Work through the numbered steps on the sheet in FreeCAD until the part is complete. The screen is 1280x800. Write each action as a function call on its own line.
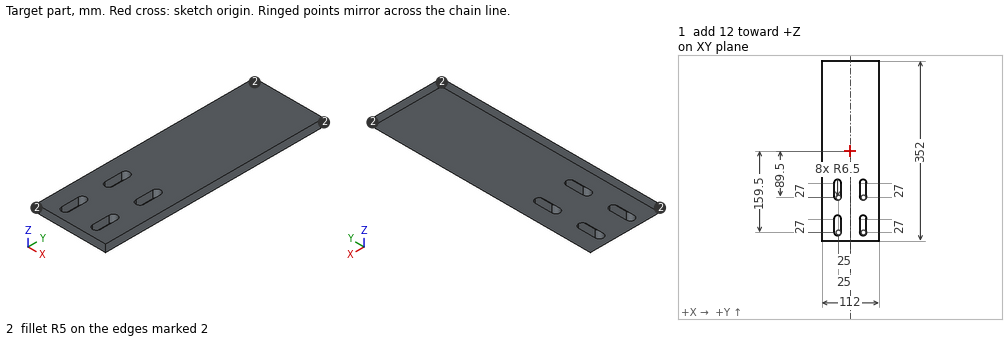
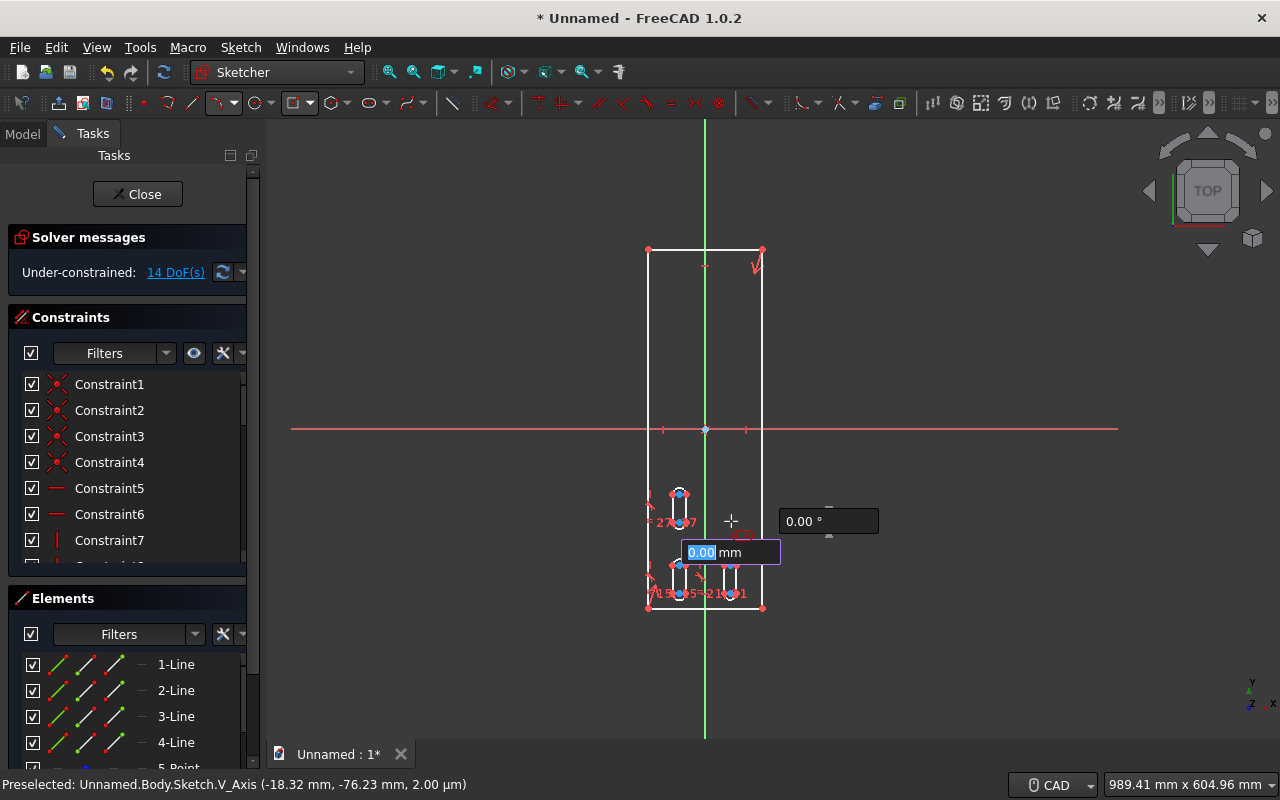
click(731, 493)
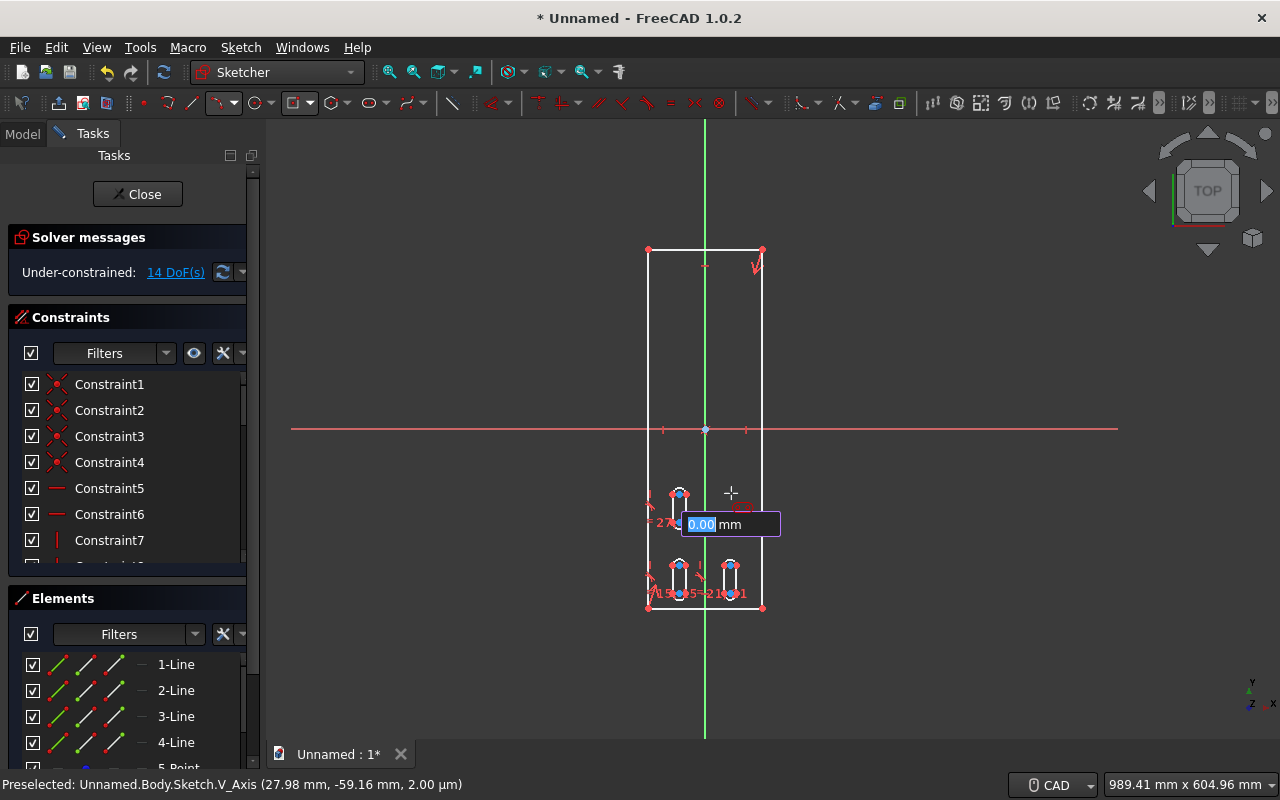
scroll(737, 507, up, 5)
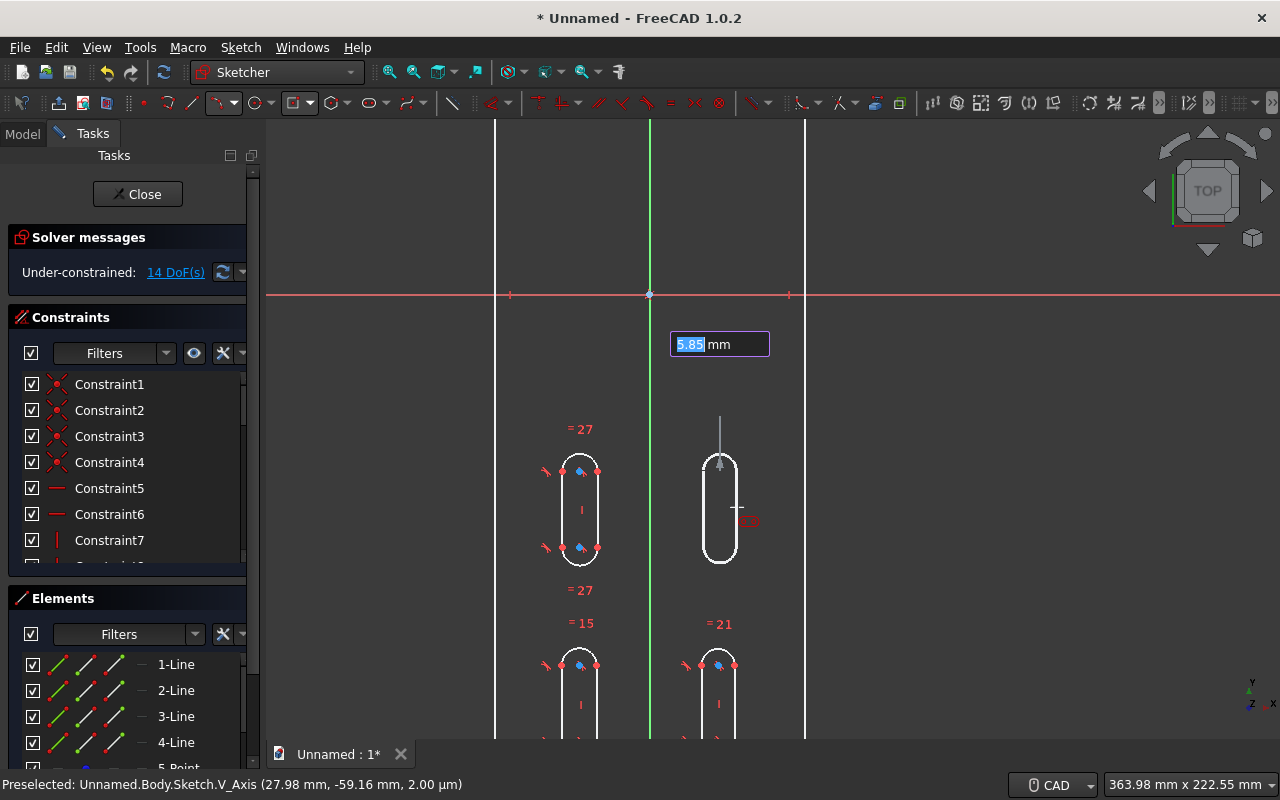
click(737, 506)
key(Escape)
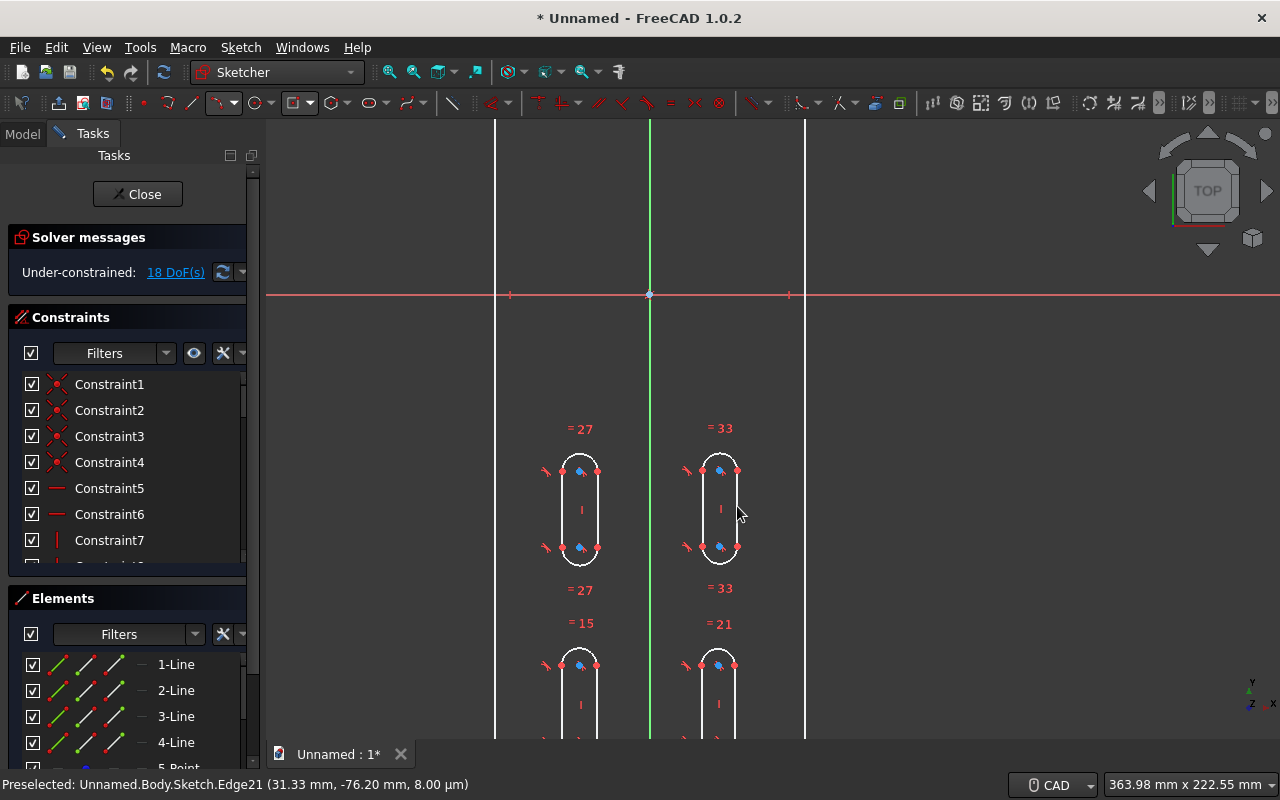
scroll(736, 507, down, 5)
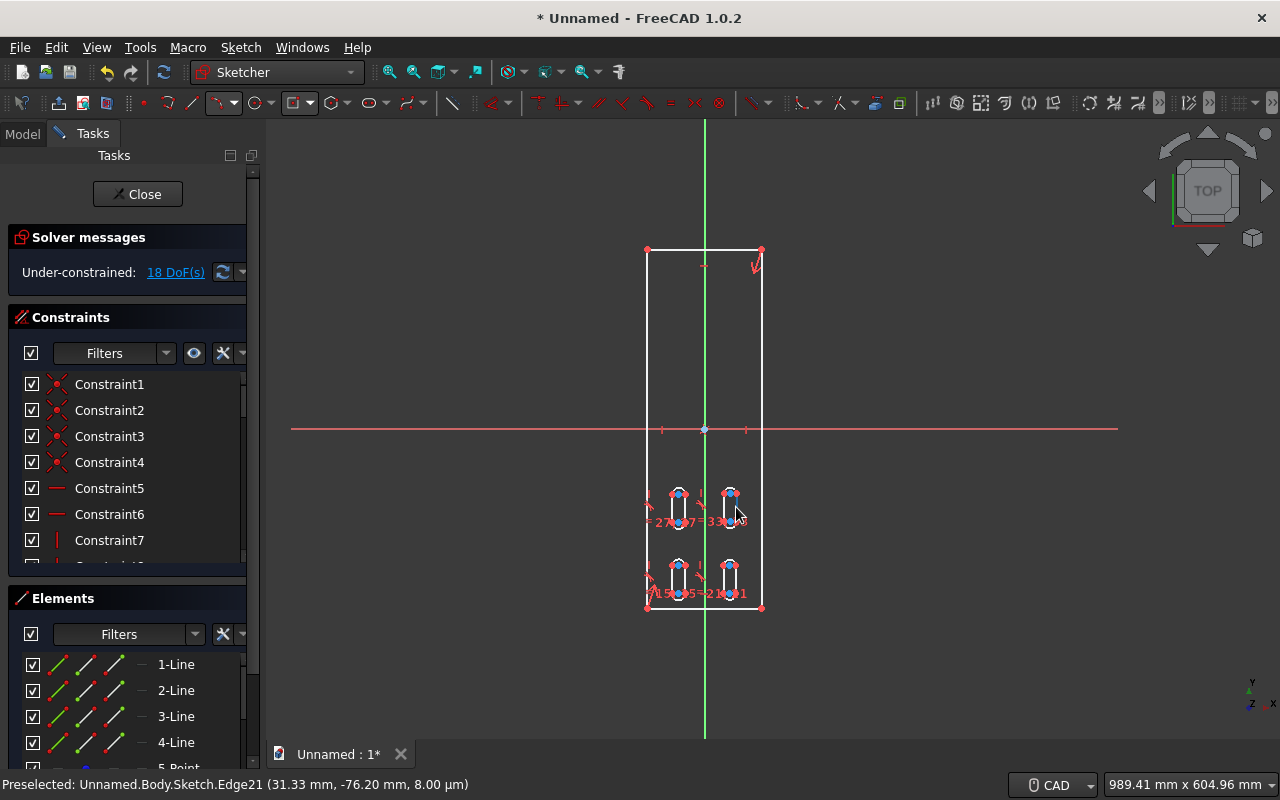
scroll(675, 599, up, 5)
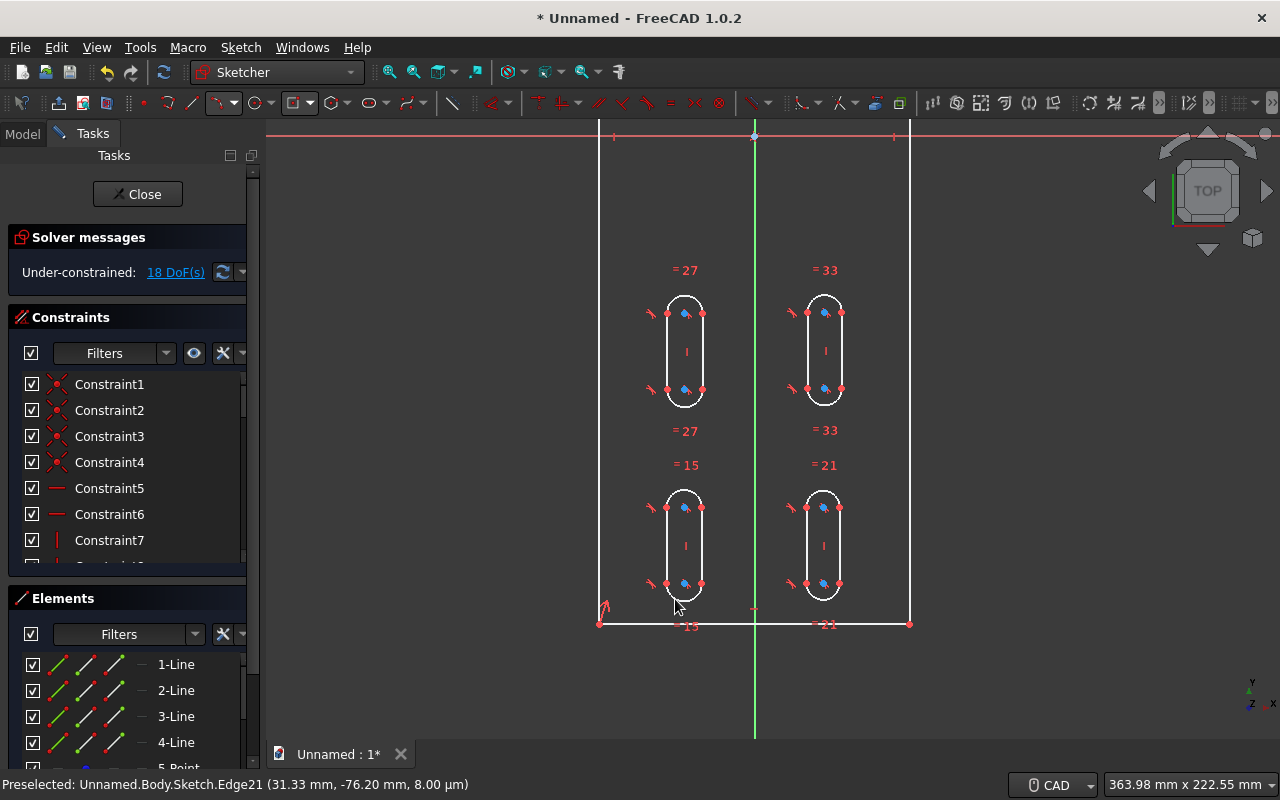
click(674, 598)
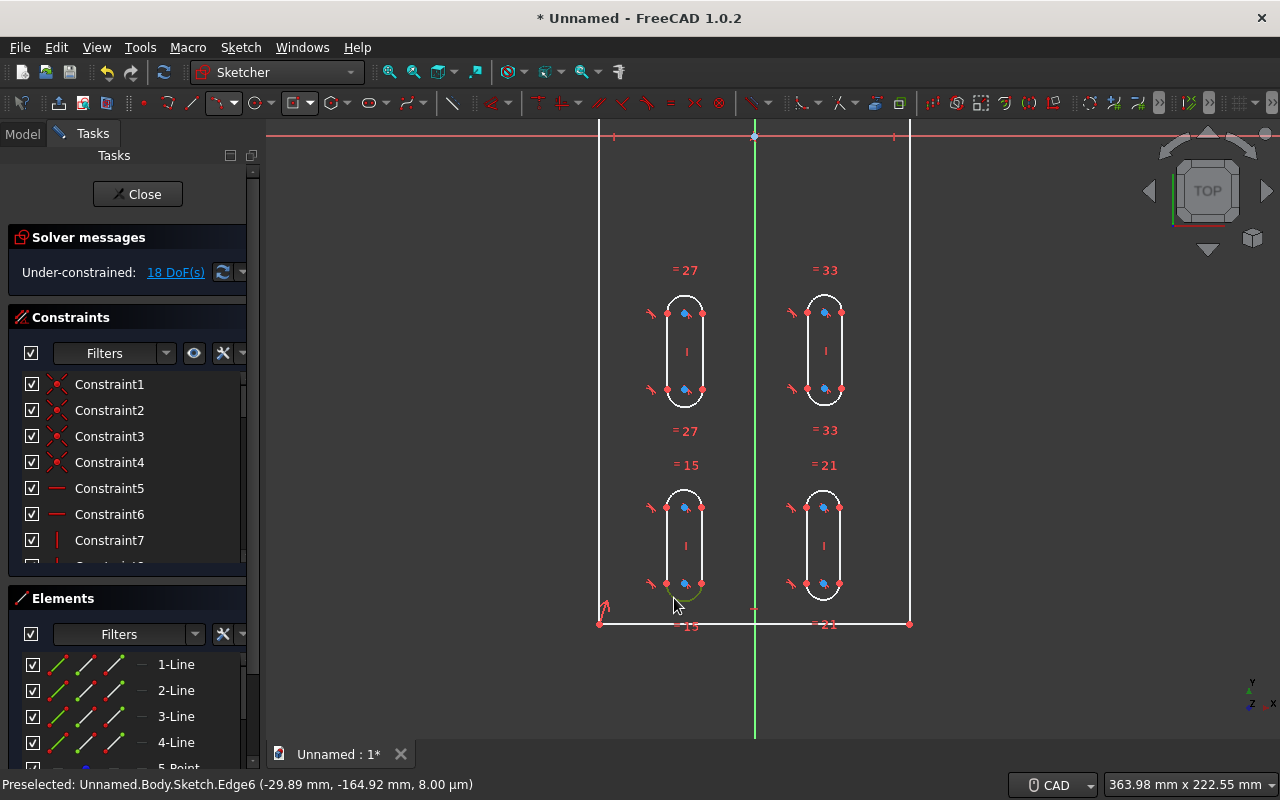
click(813, 597)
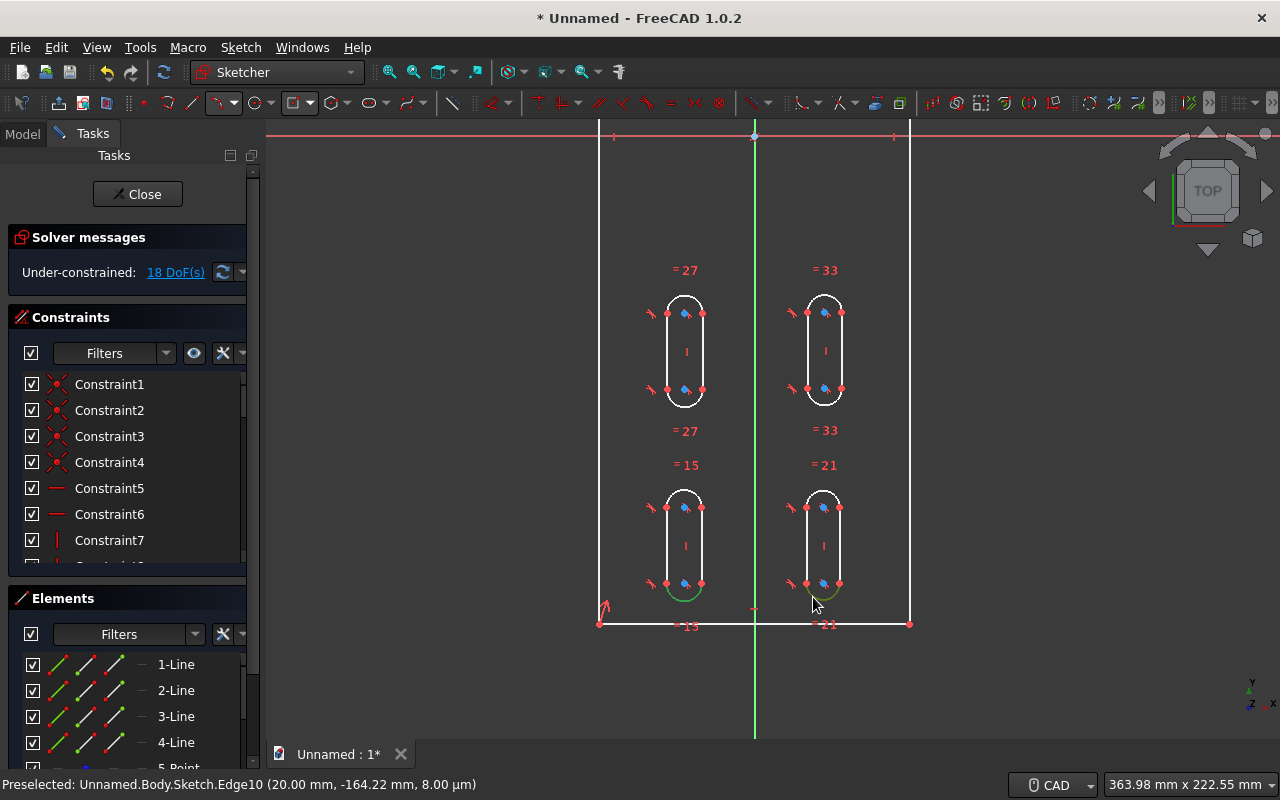
click(674, 404)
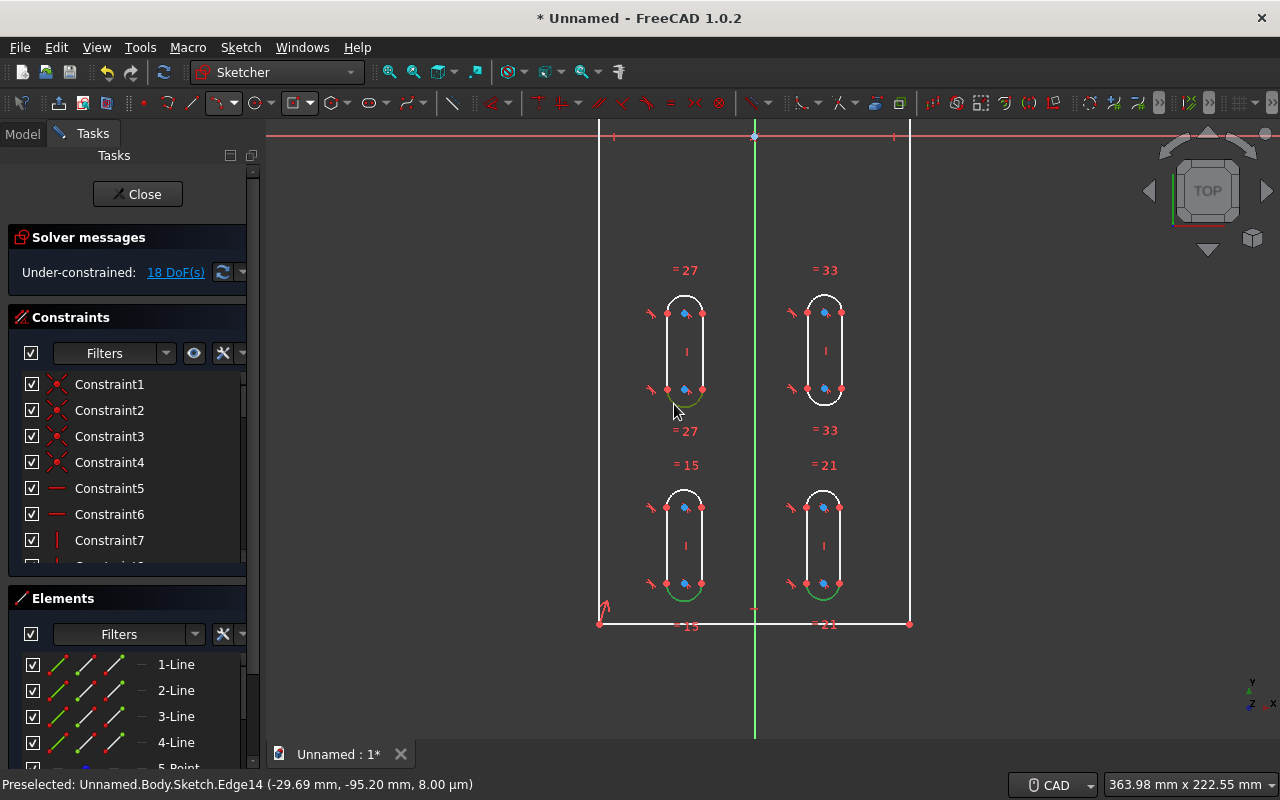
click(815, 402)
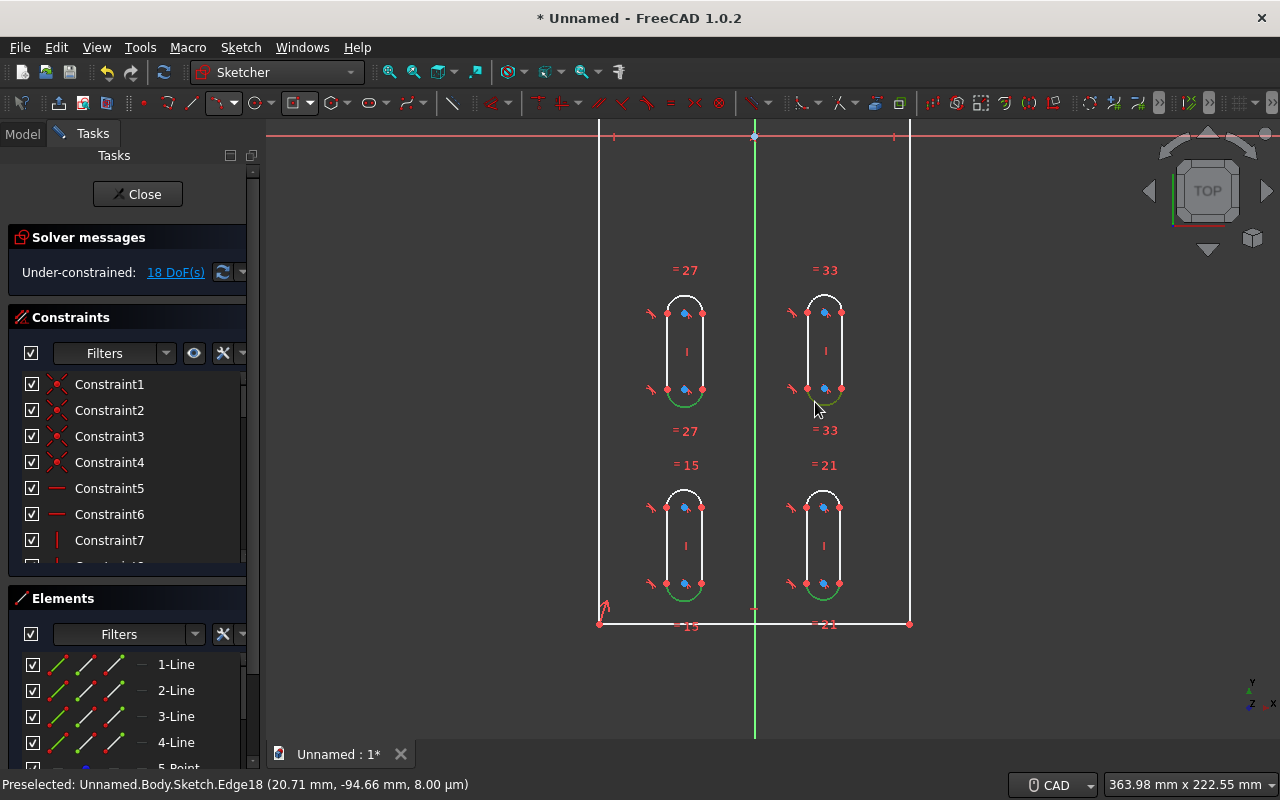
click(672, 104)